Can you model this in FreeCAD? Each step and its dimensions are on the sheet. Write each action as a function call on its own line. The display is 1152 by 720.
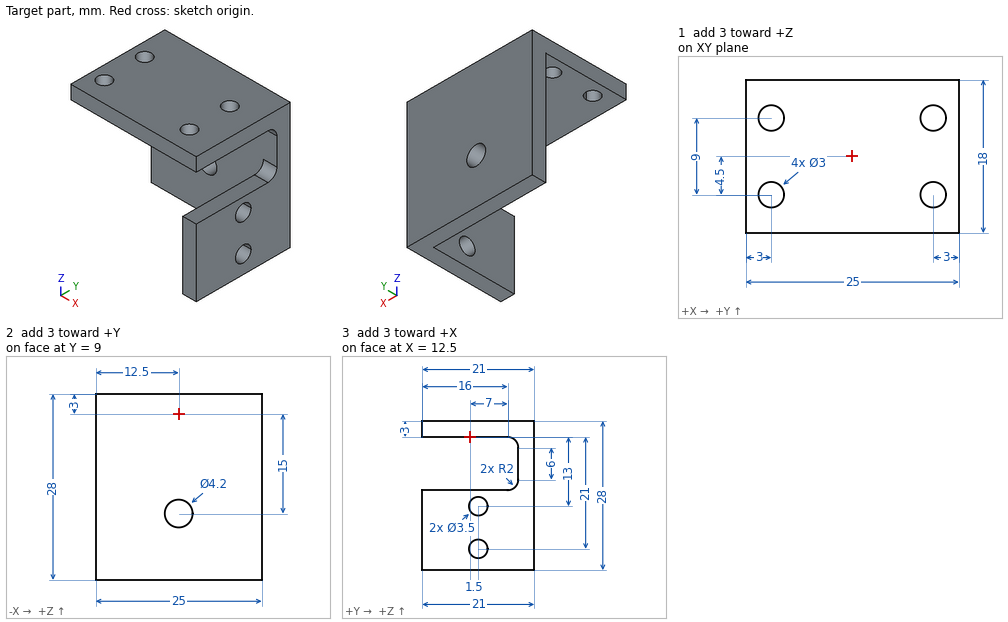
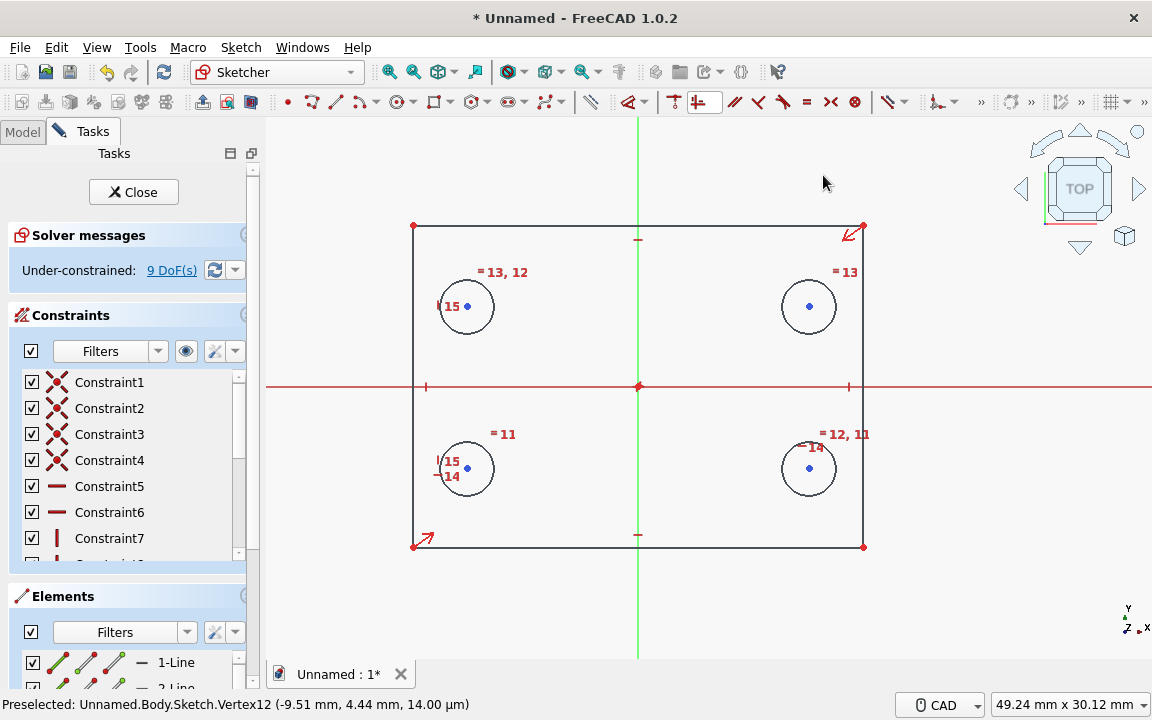
click(809, 469)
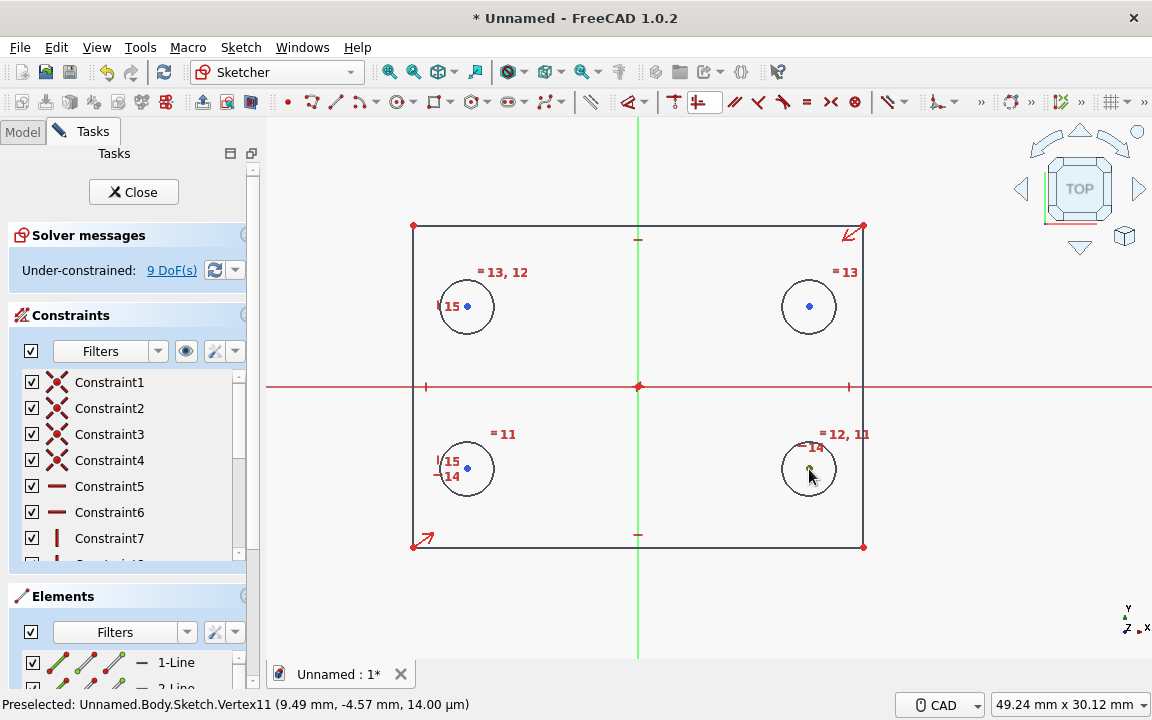
click(809, 307)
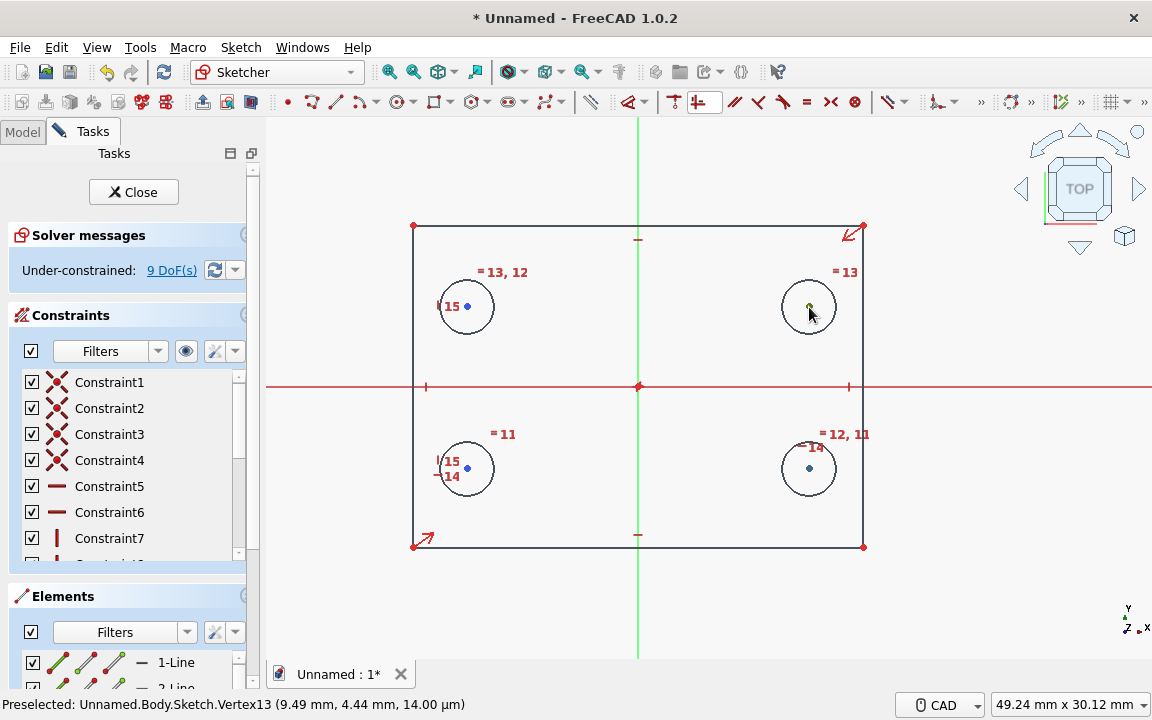
key(v)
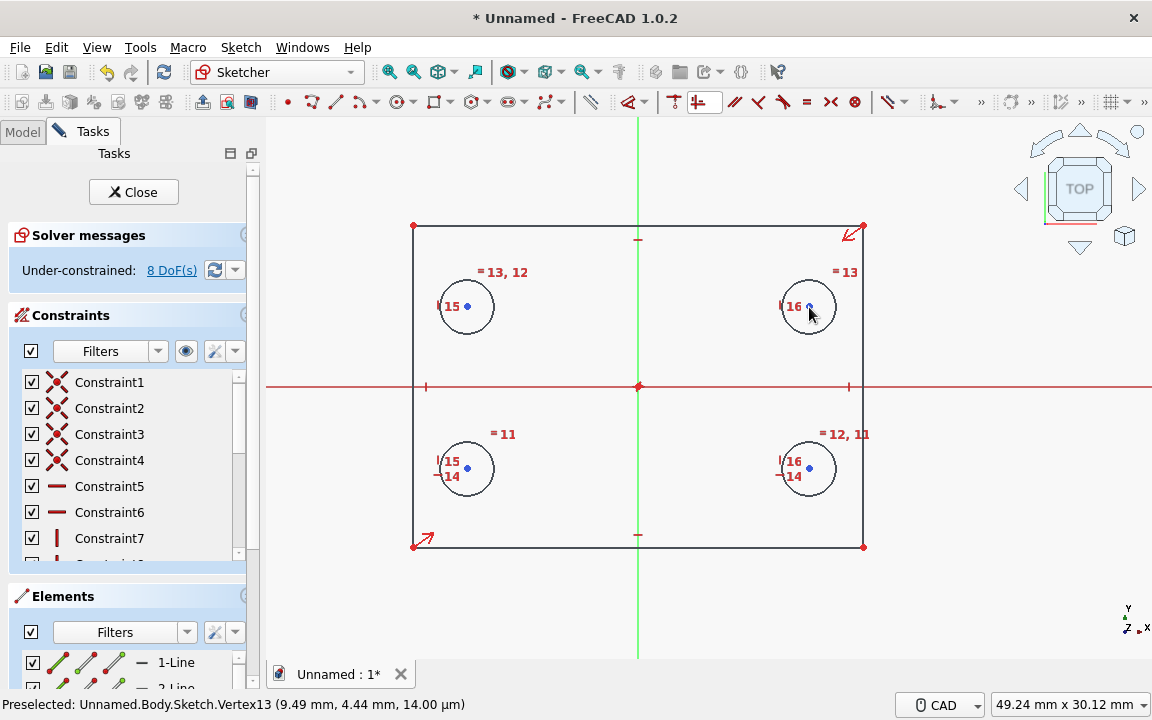
click(467, 307)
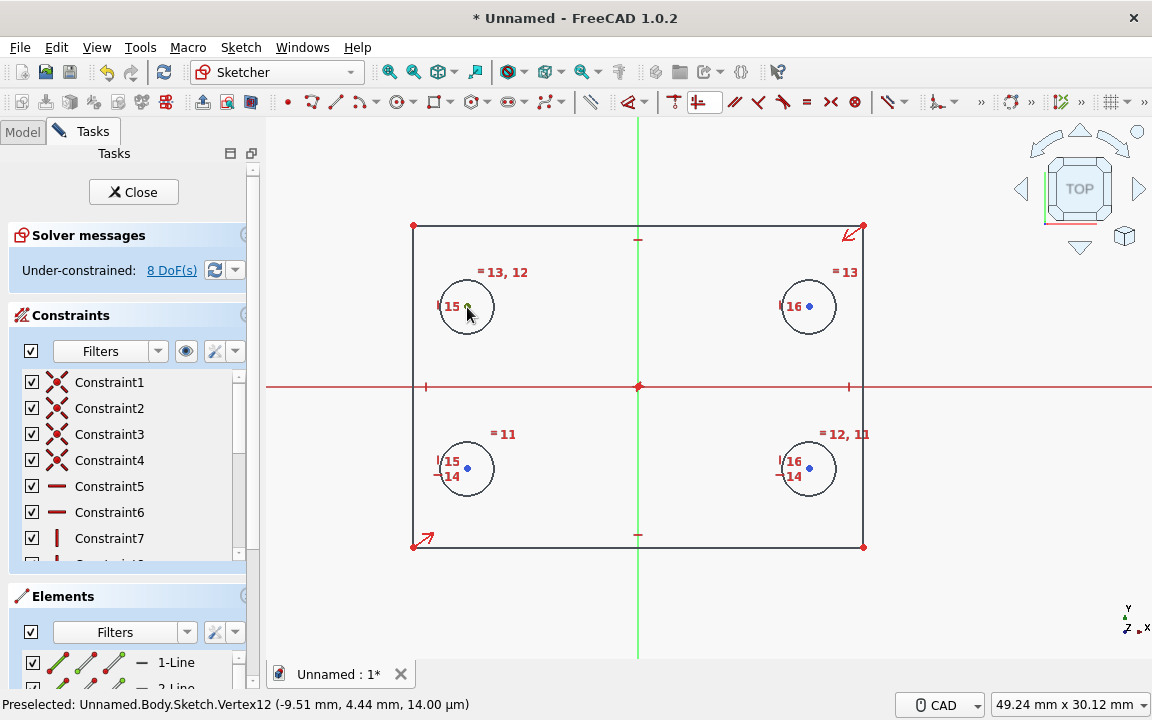
click(809, 307)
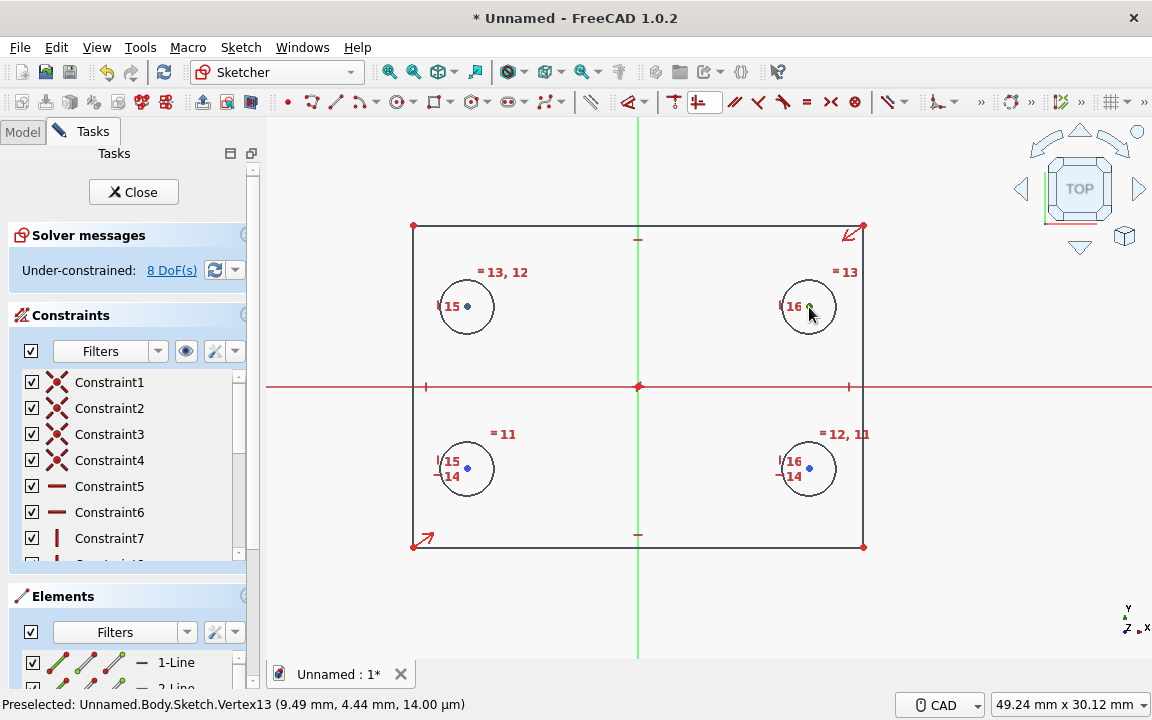
key(h)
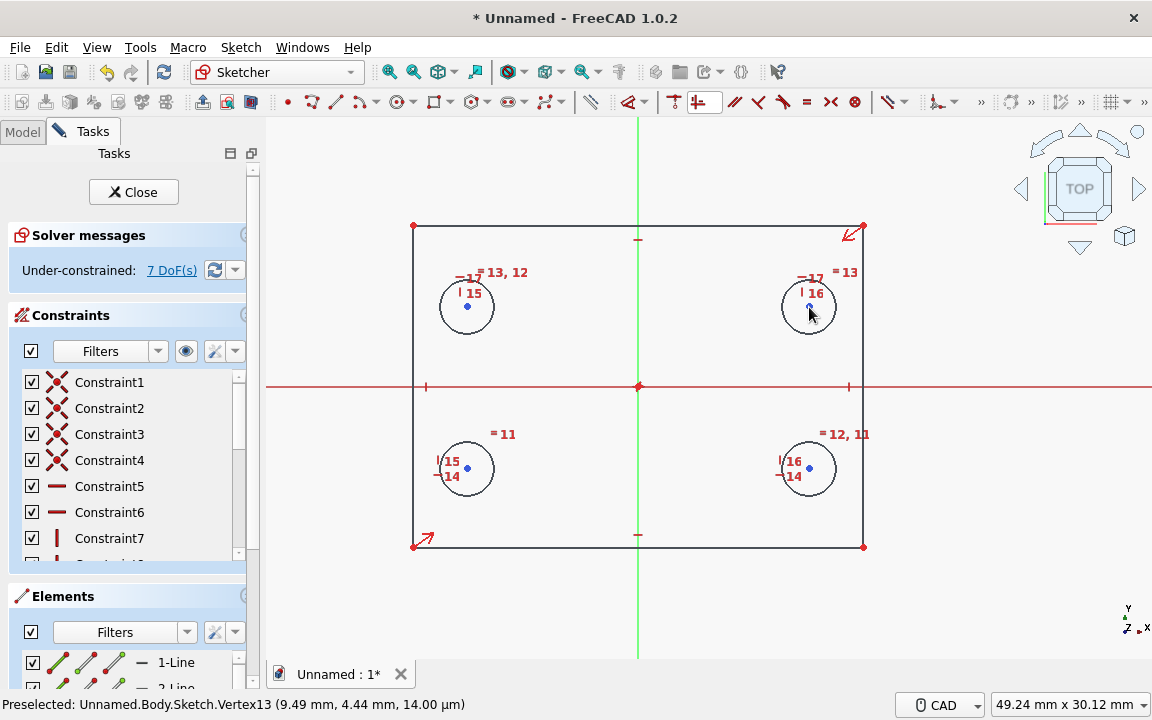
click(486, 450)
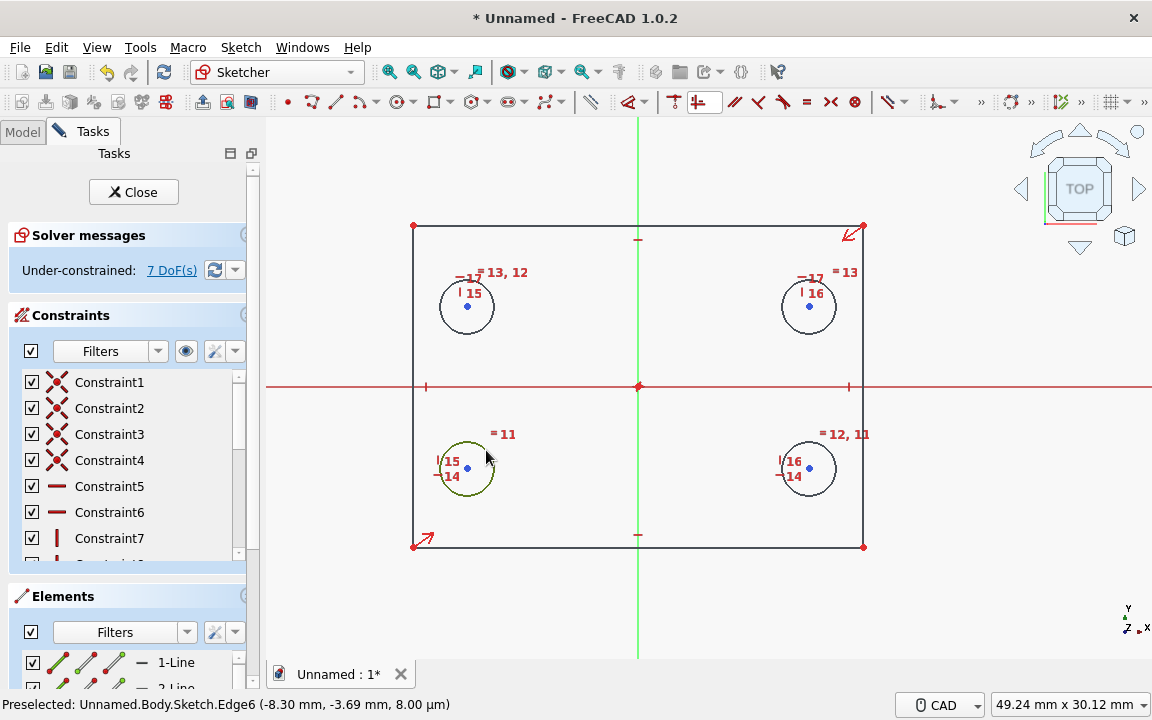
key(k)
key(o)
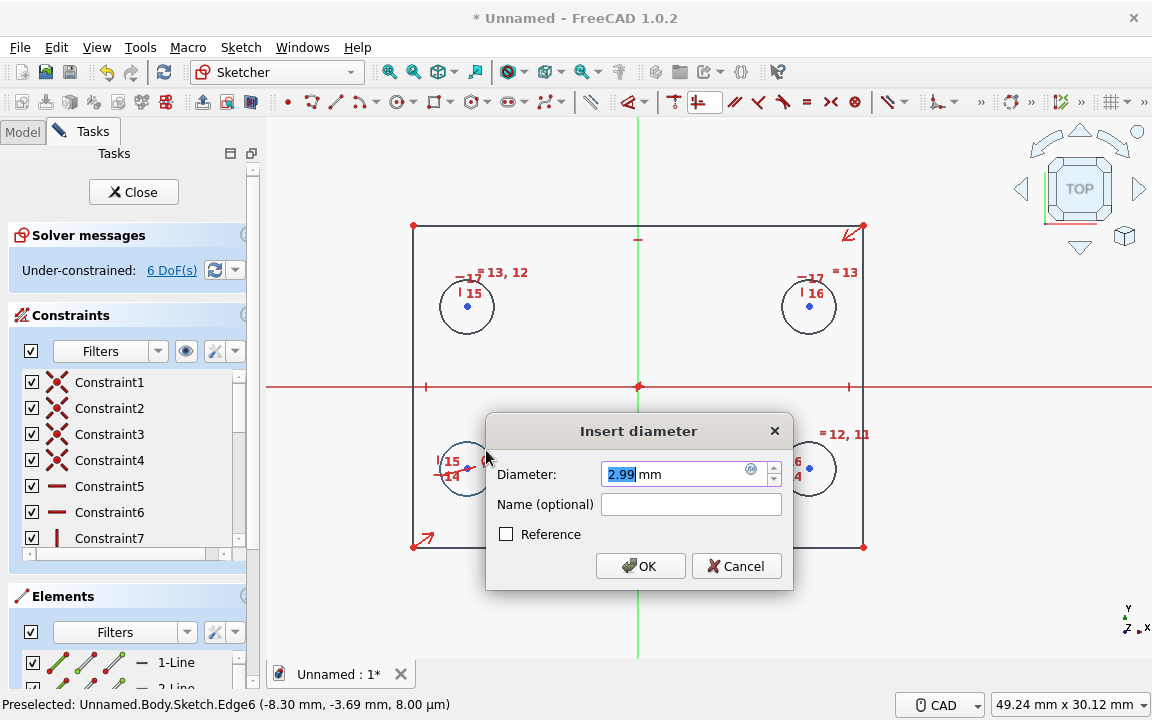
text(3)
key(Return)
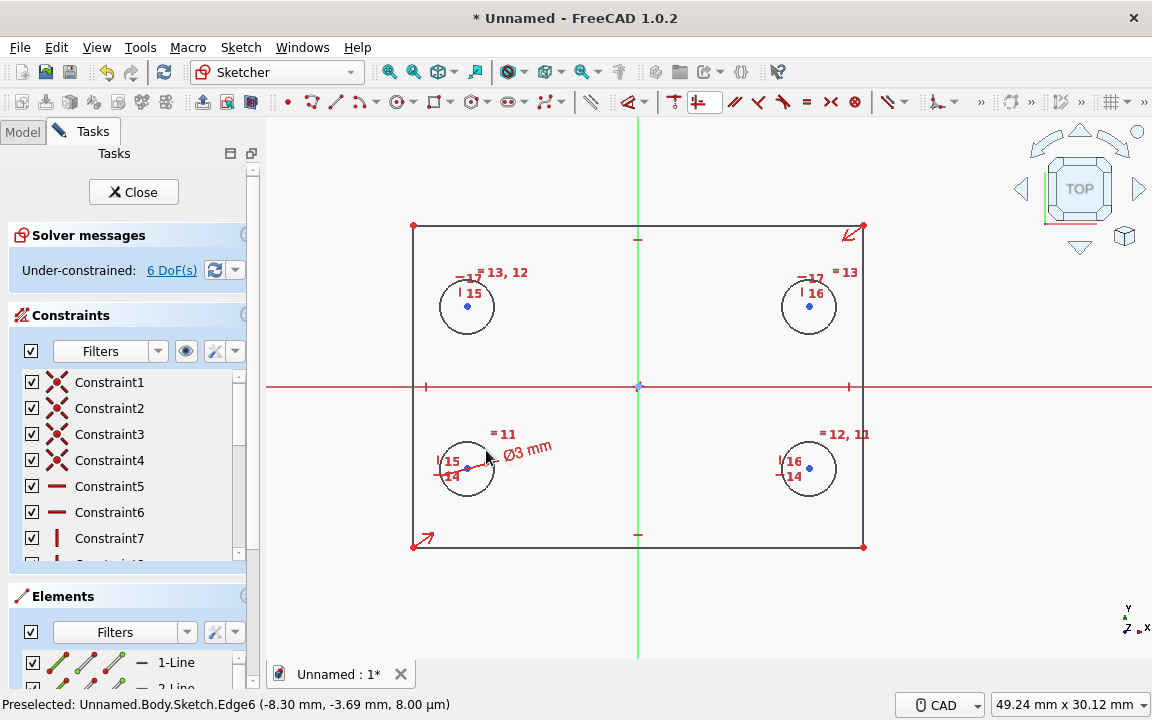
click(548, 548)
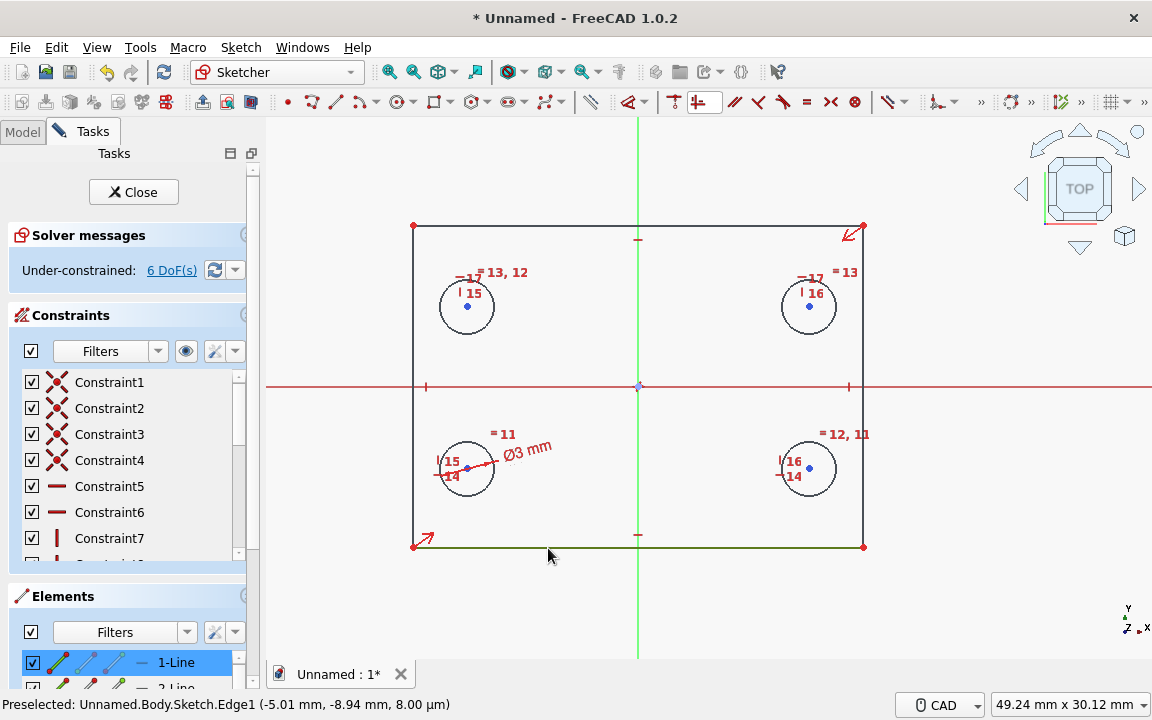
key(l)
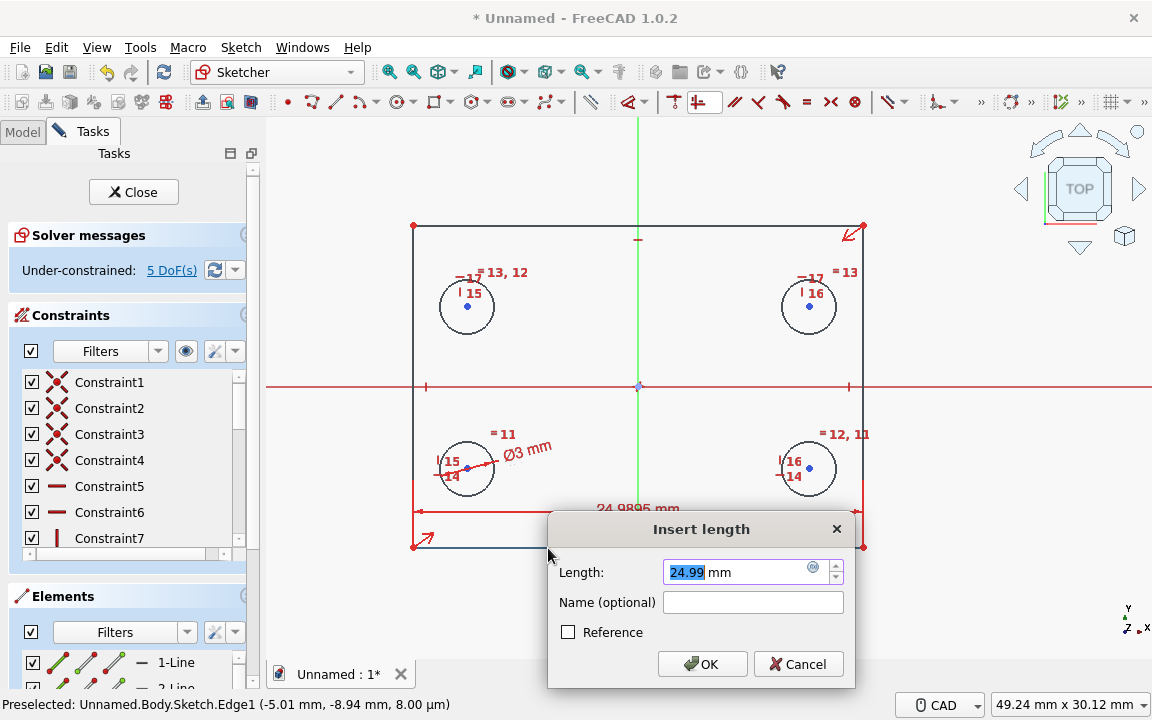
text(25)
key(Return)